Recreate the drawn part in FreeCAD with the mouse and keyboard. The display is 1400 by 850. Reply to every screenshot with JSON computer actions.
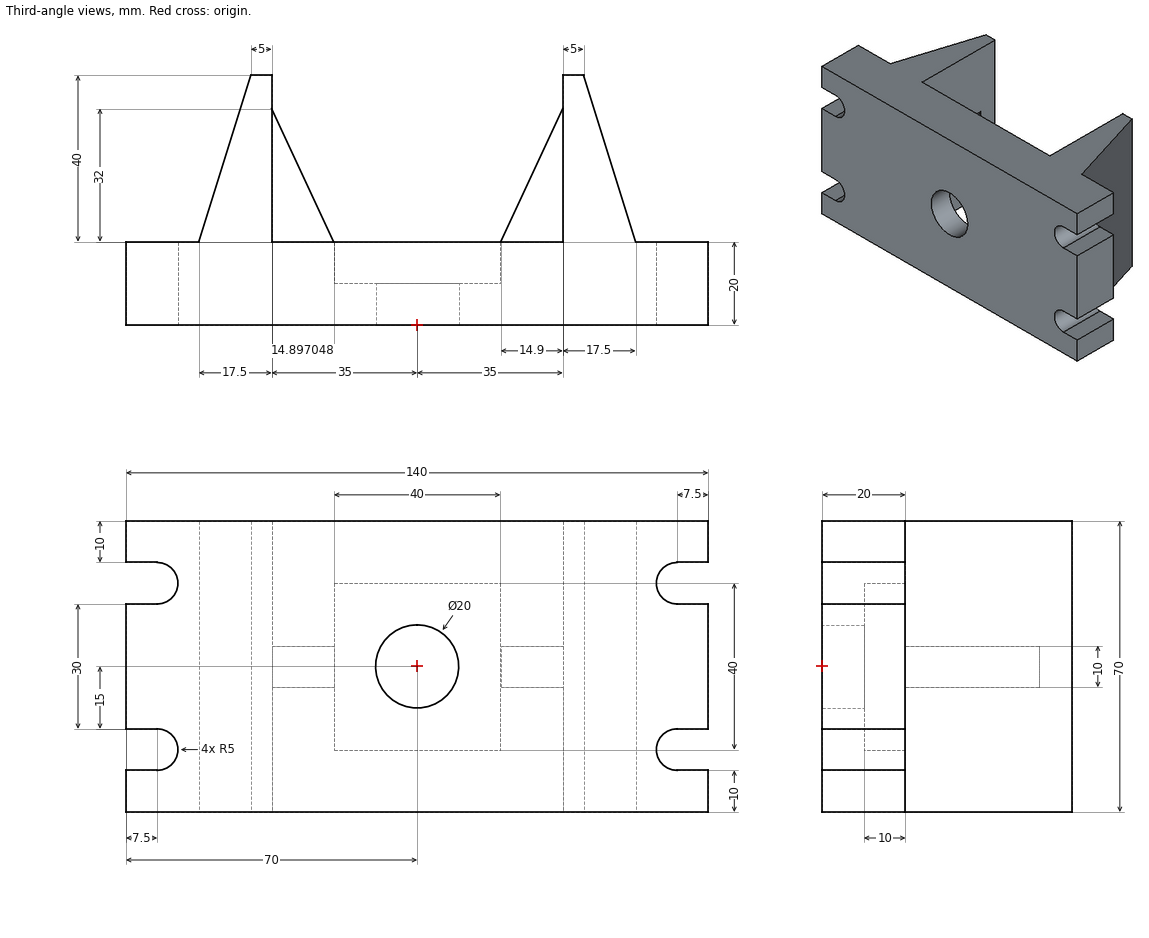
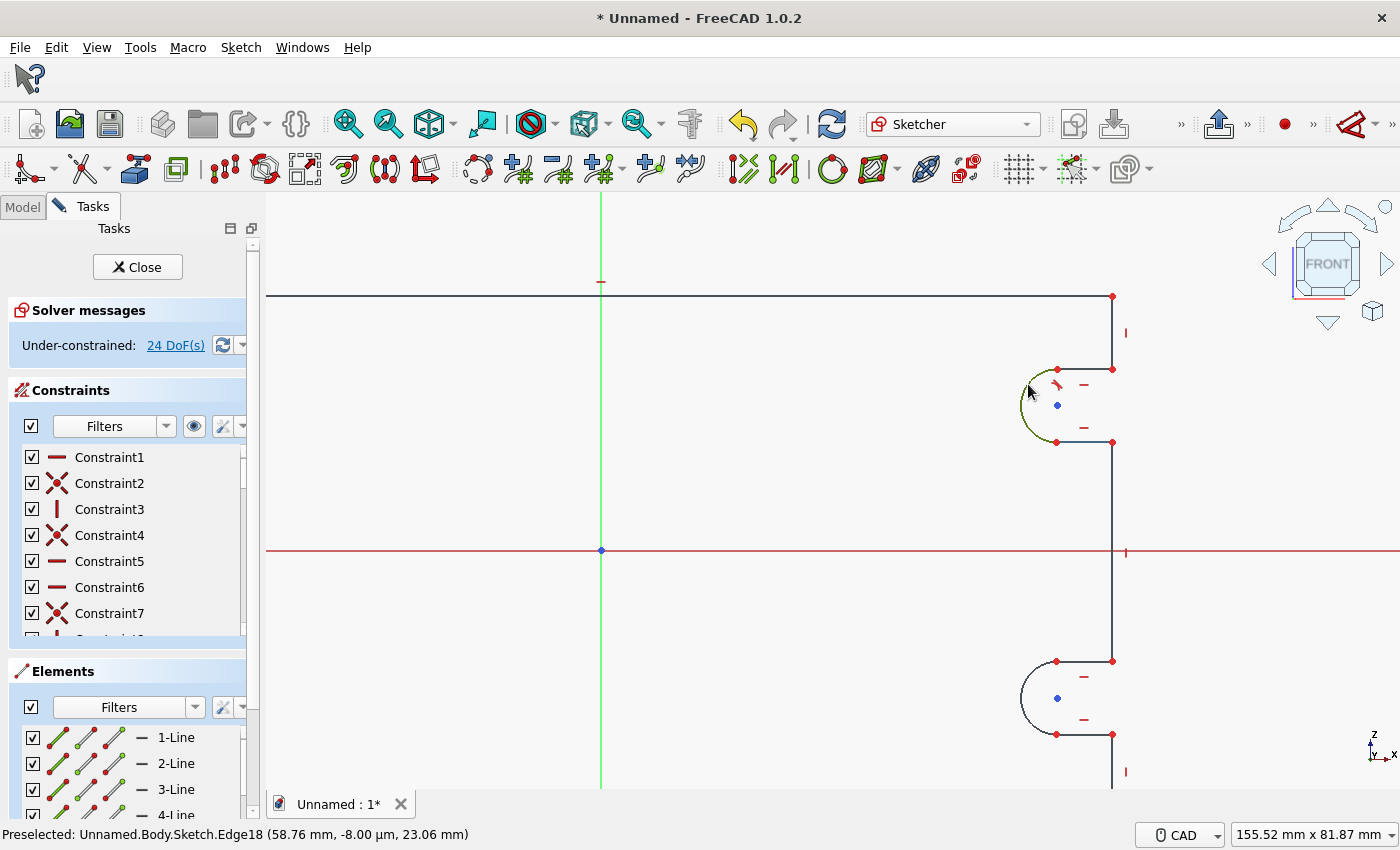
{"action": "key", "text": "t"}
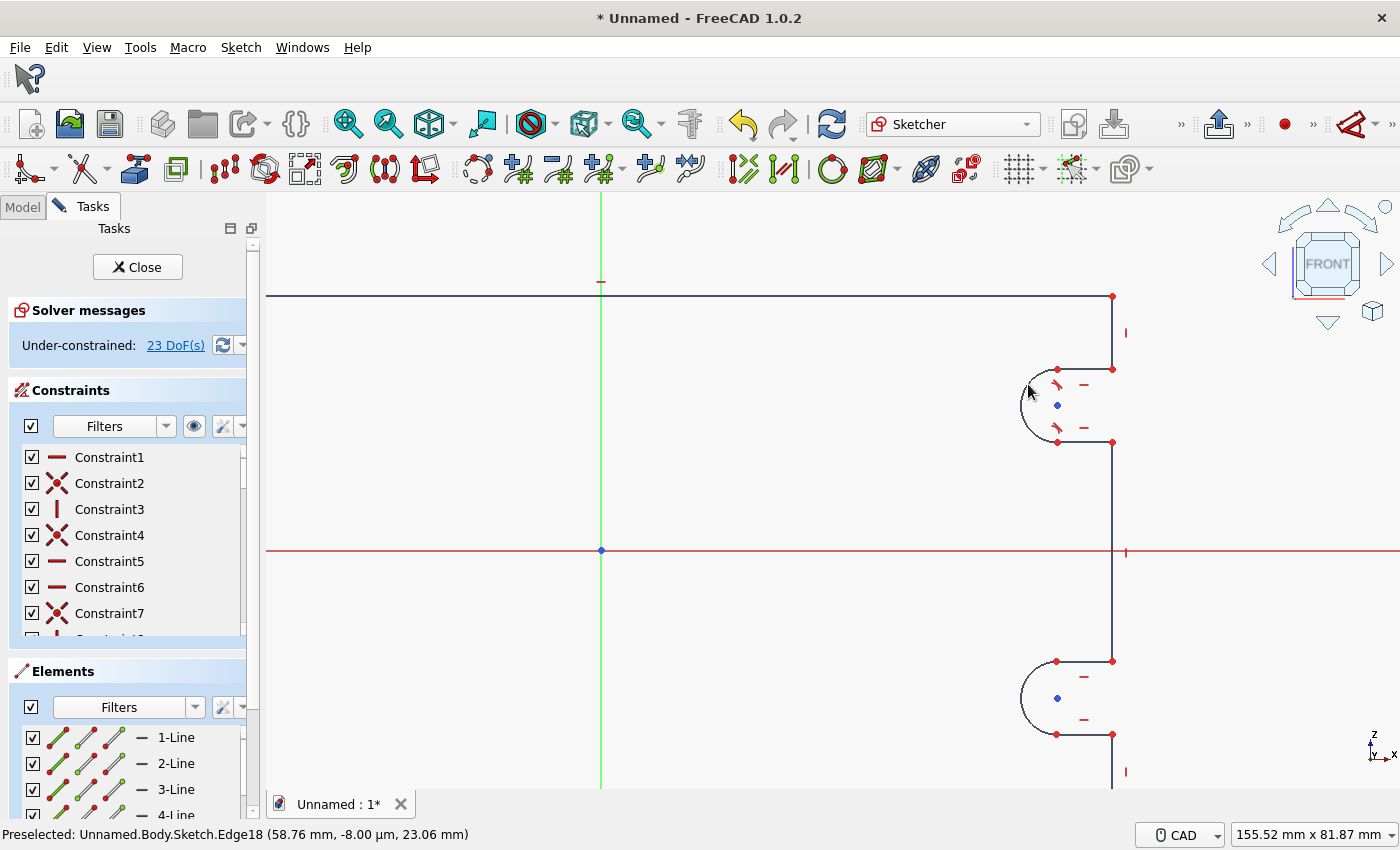
{"action": "left_click", "coordinate": [1095, 662]}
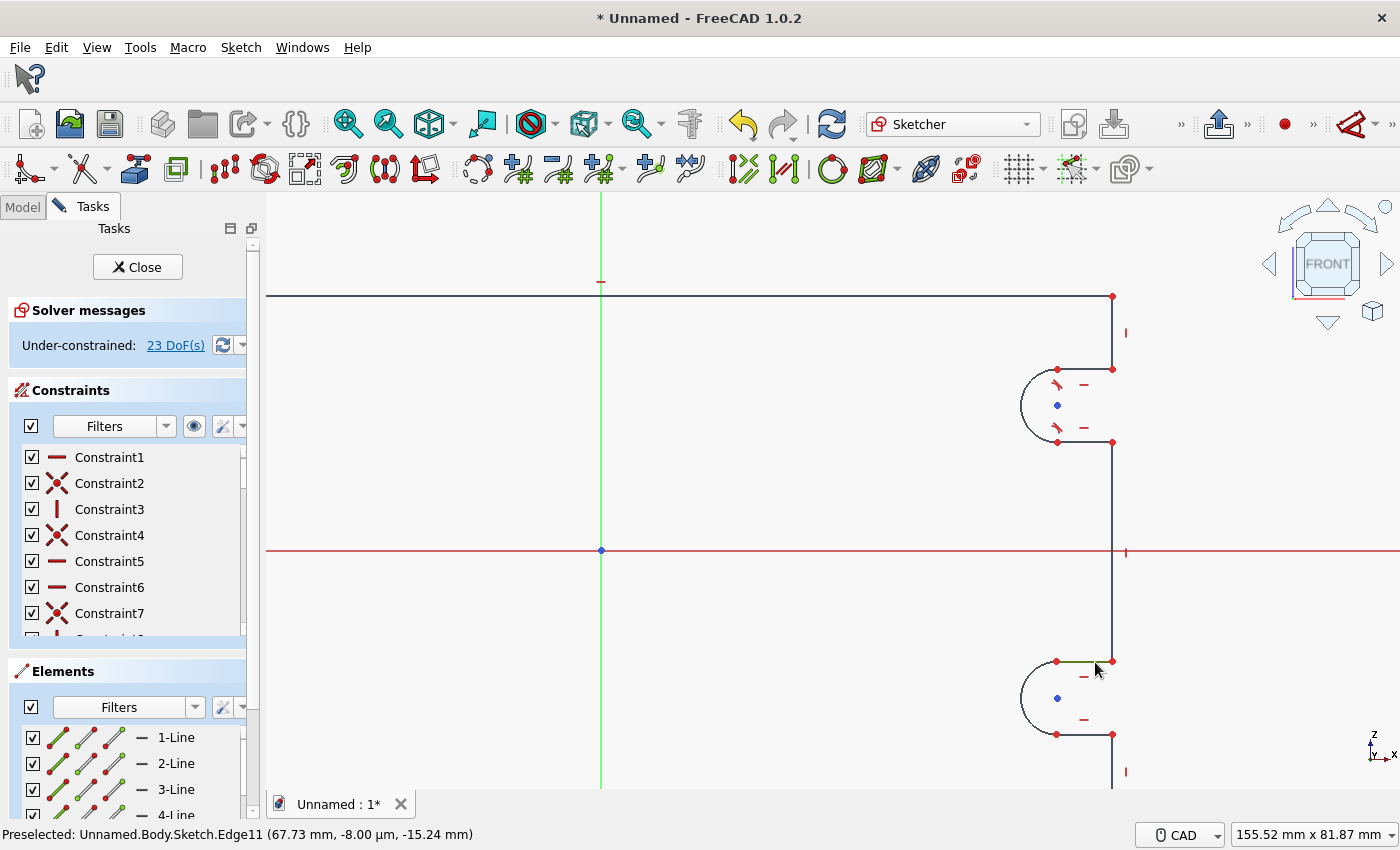
{"action": "left_click", "coordinate": [1028, 677]}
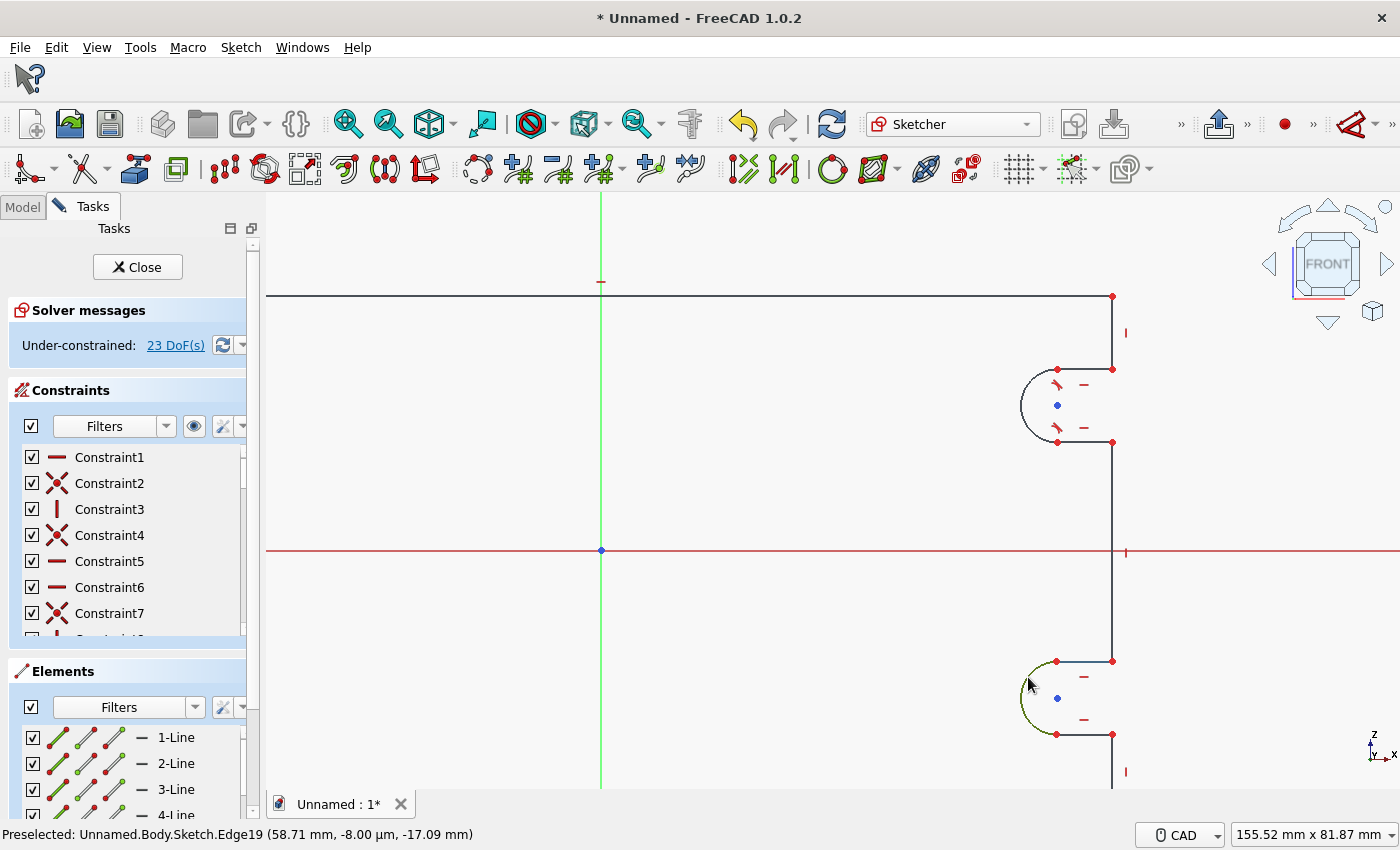
{"action": "key", "text": "t"}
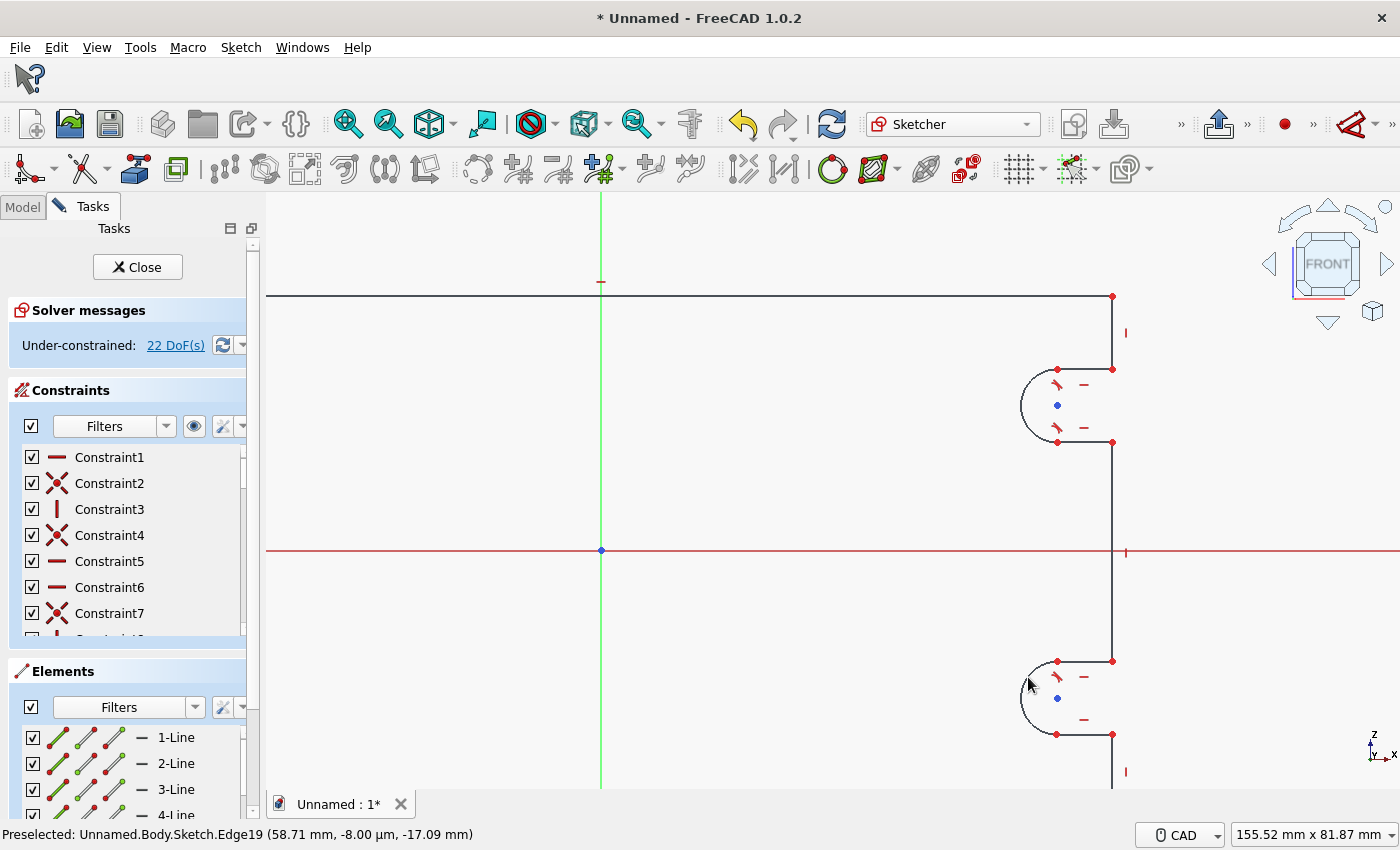
{"action": "left_click", "coordinate": [1073, 735]}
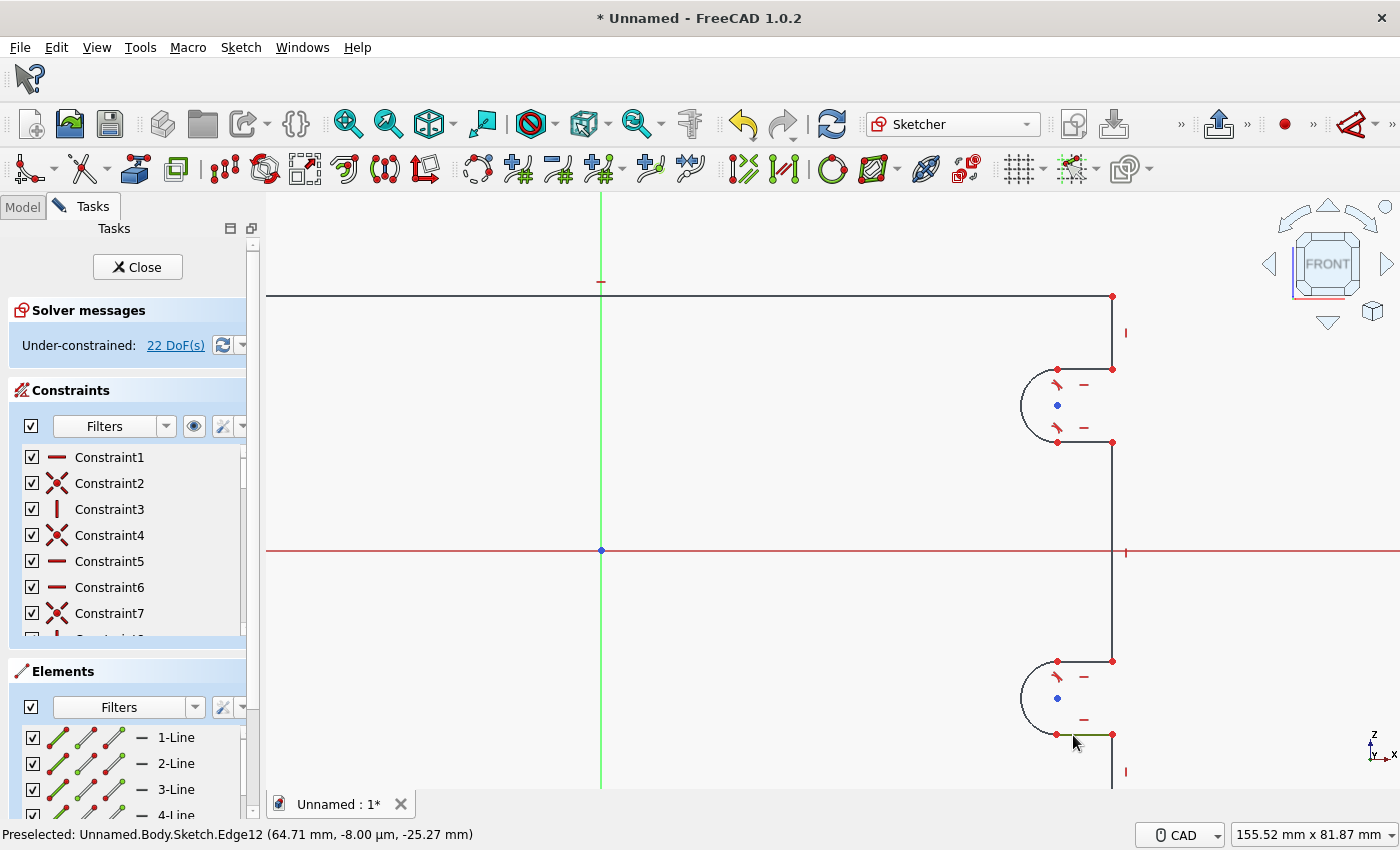
{"action": "left_click", "coordinate": [1028, 677]}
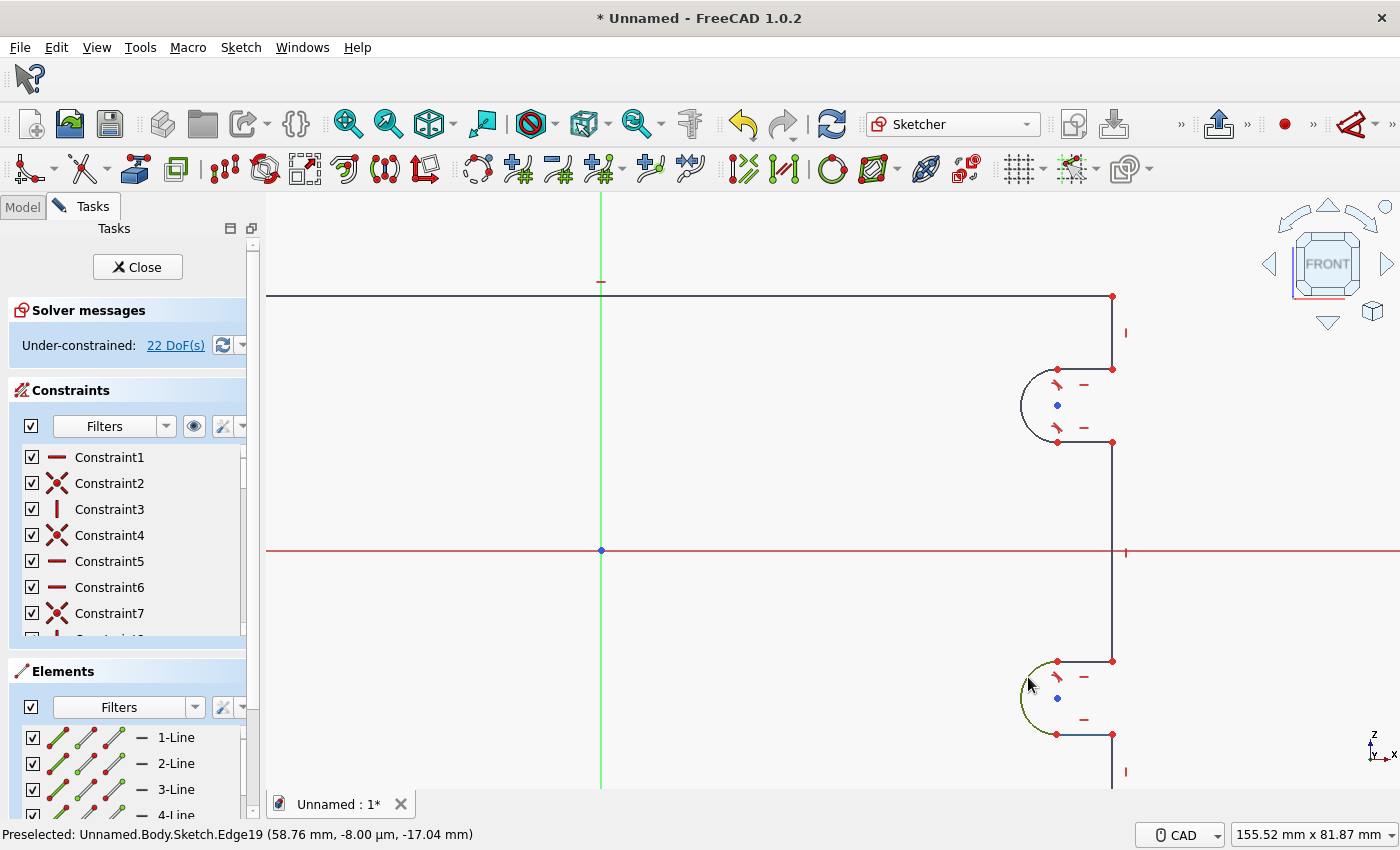
{"action": "key", "text": "t"}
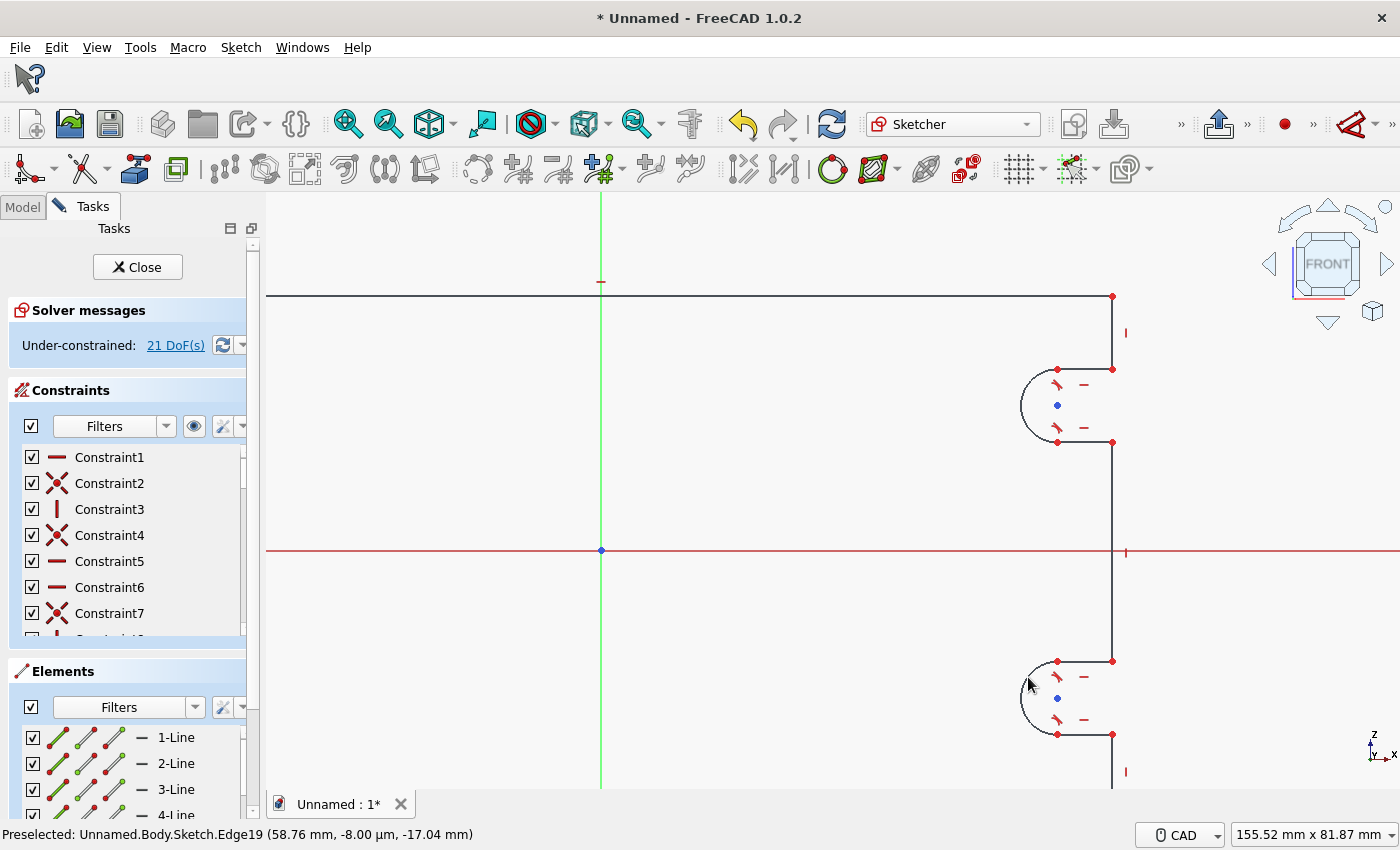
{"action": "scroll", "coordinate": [1097, 368], "scroll_direction": "down", "scroll_amount": 2}